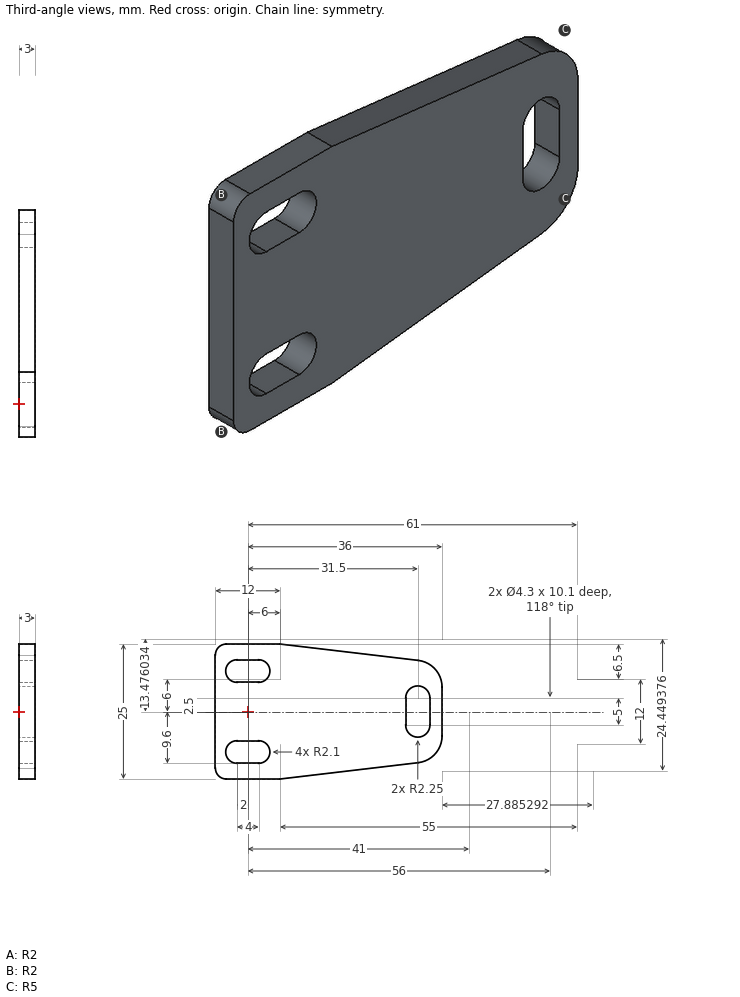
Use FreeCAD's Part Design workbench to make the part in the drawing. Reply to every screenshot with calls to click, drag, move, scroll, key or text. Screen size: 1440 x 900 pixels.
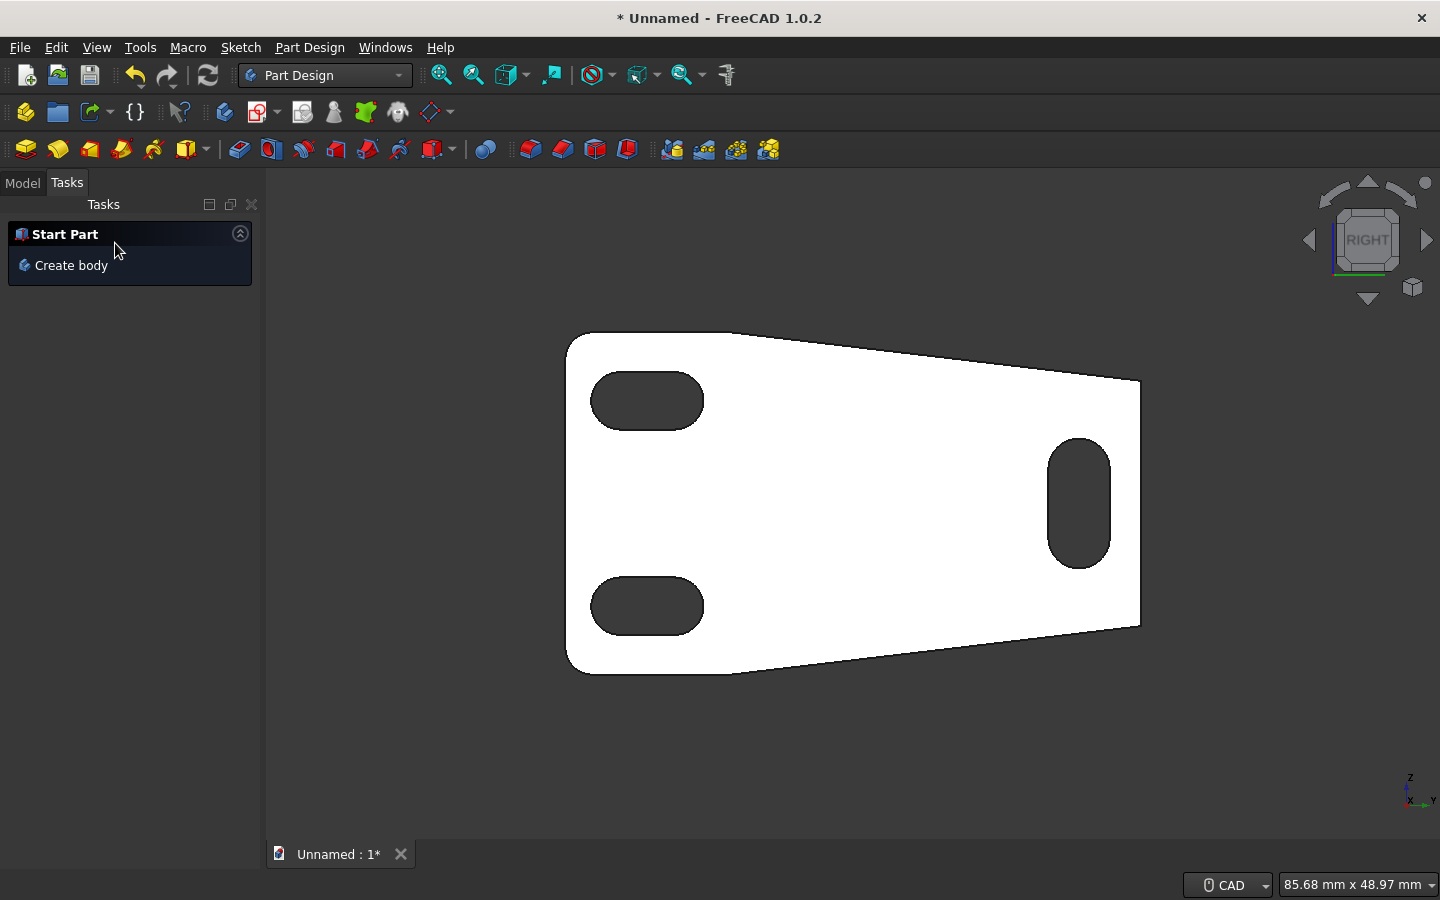
key(5)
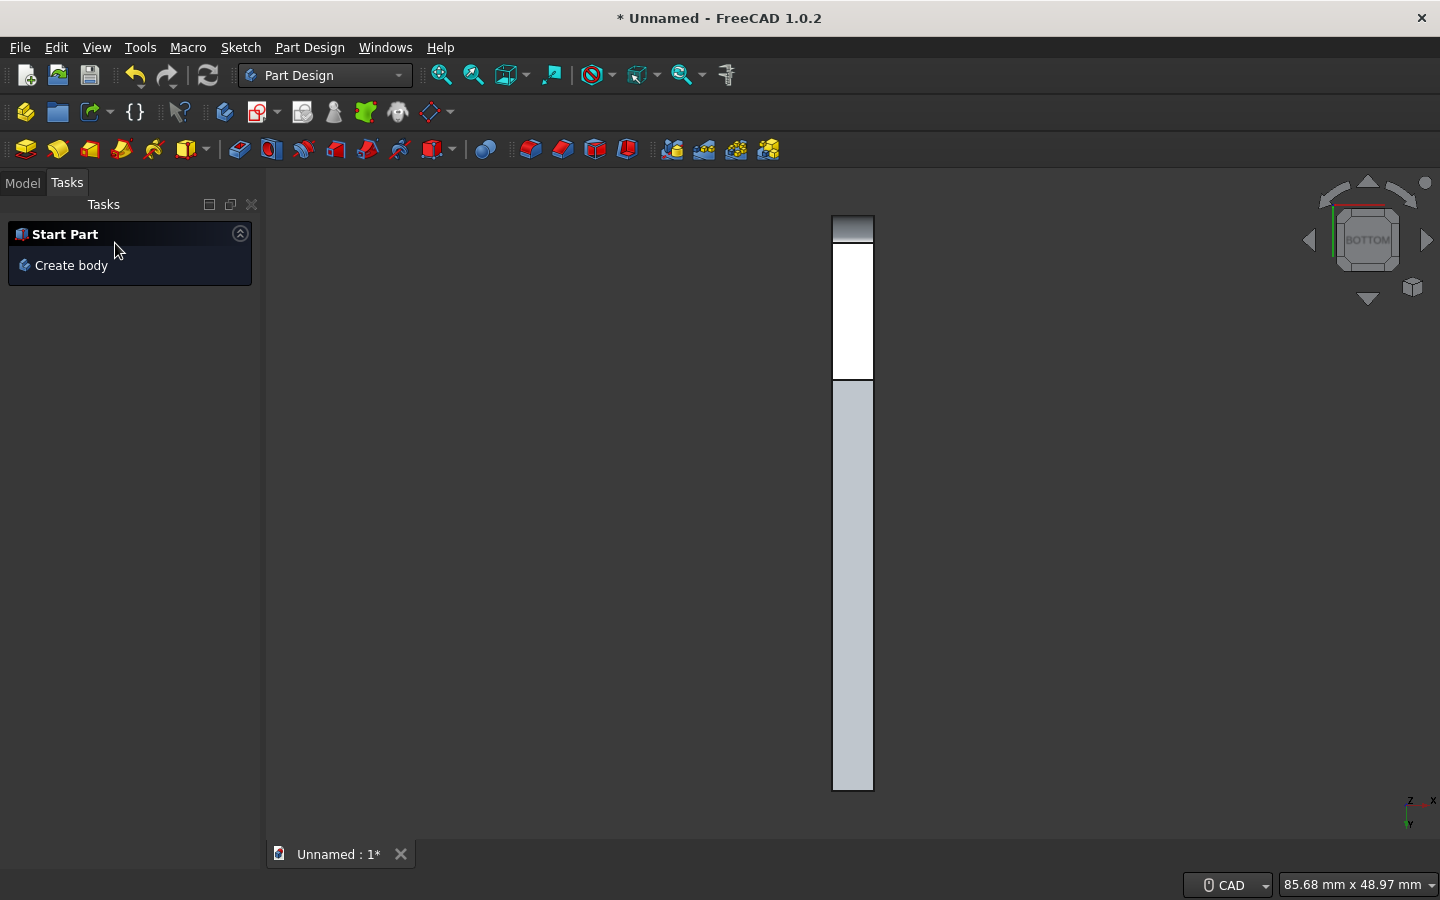
key(4)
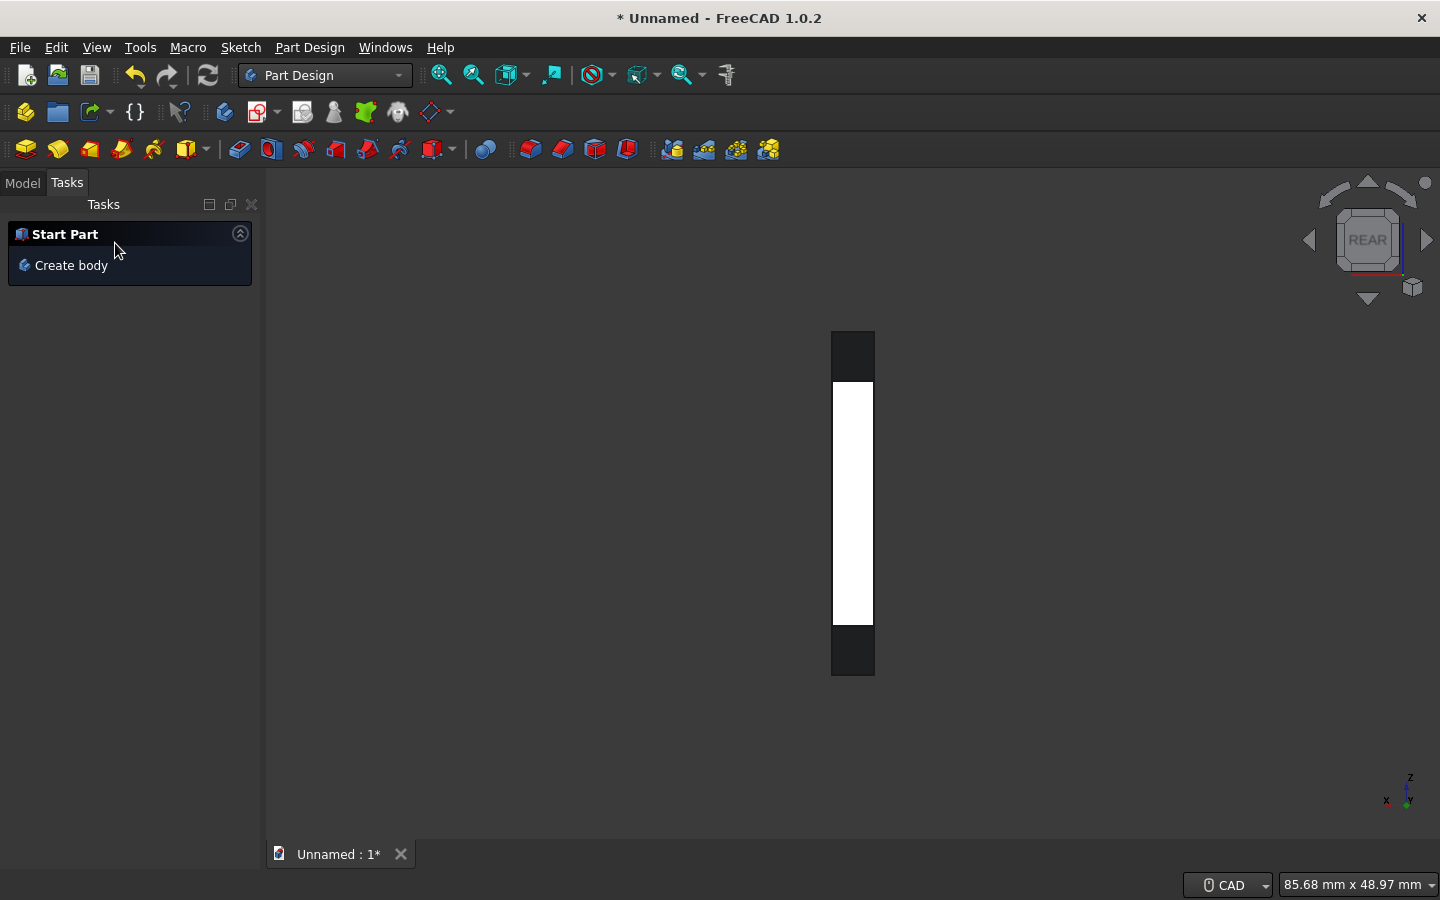
click(853, 380)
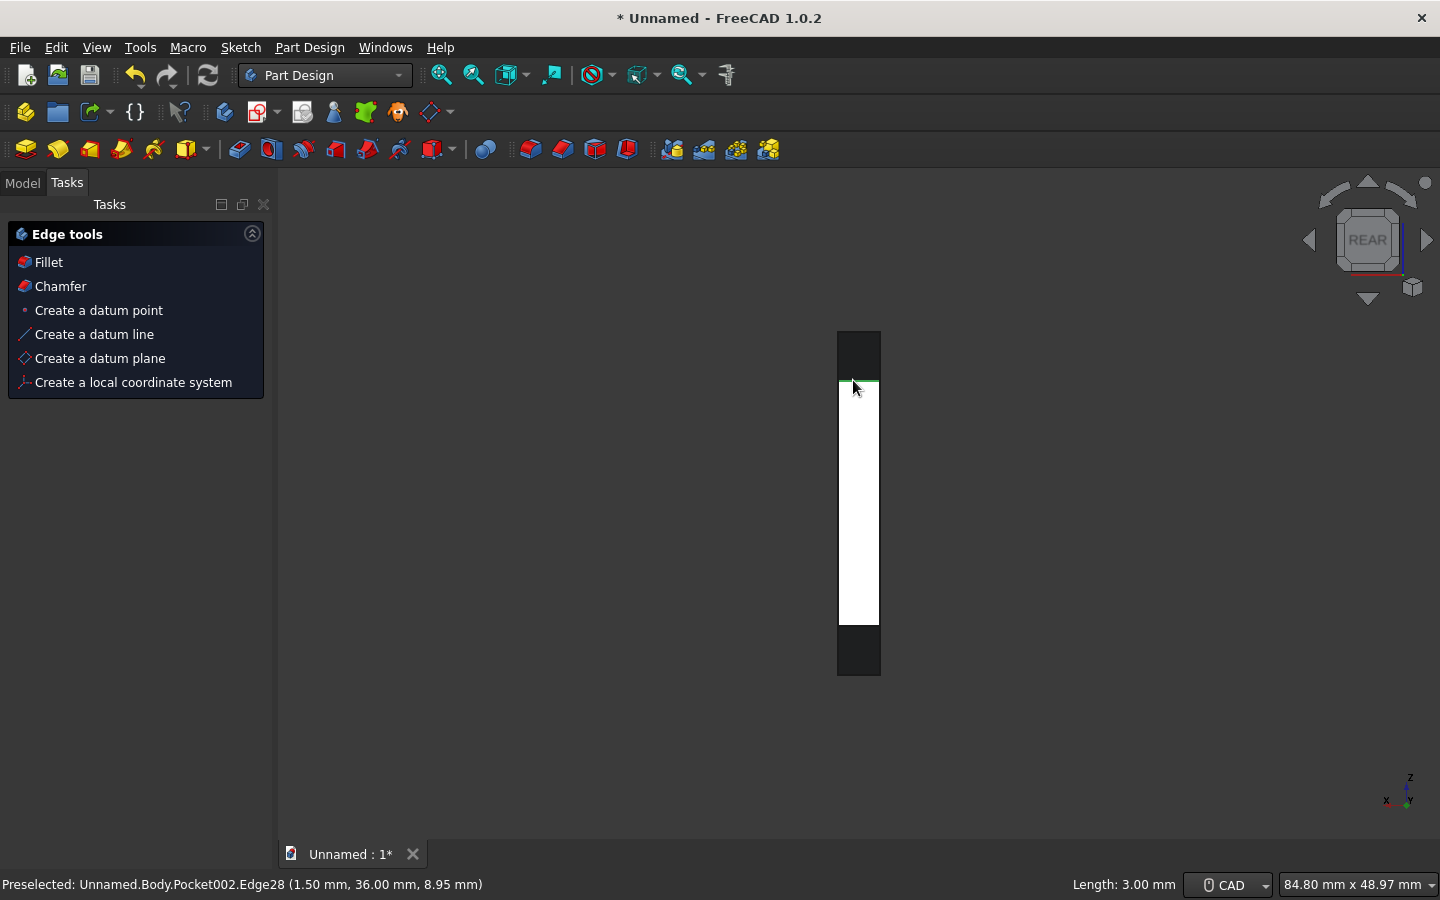
click(859, 625, ctrl)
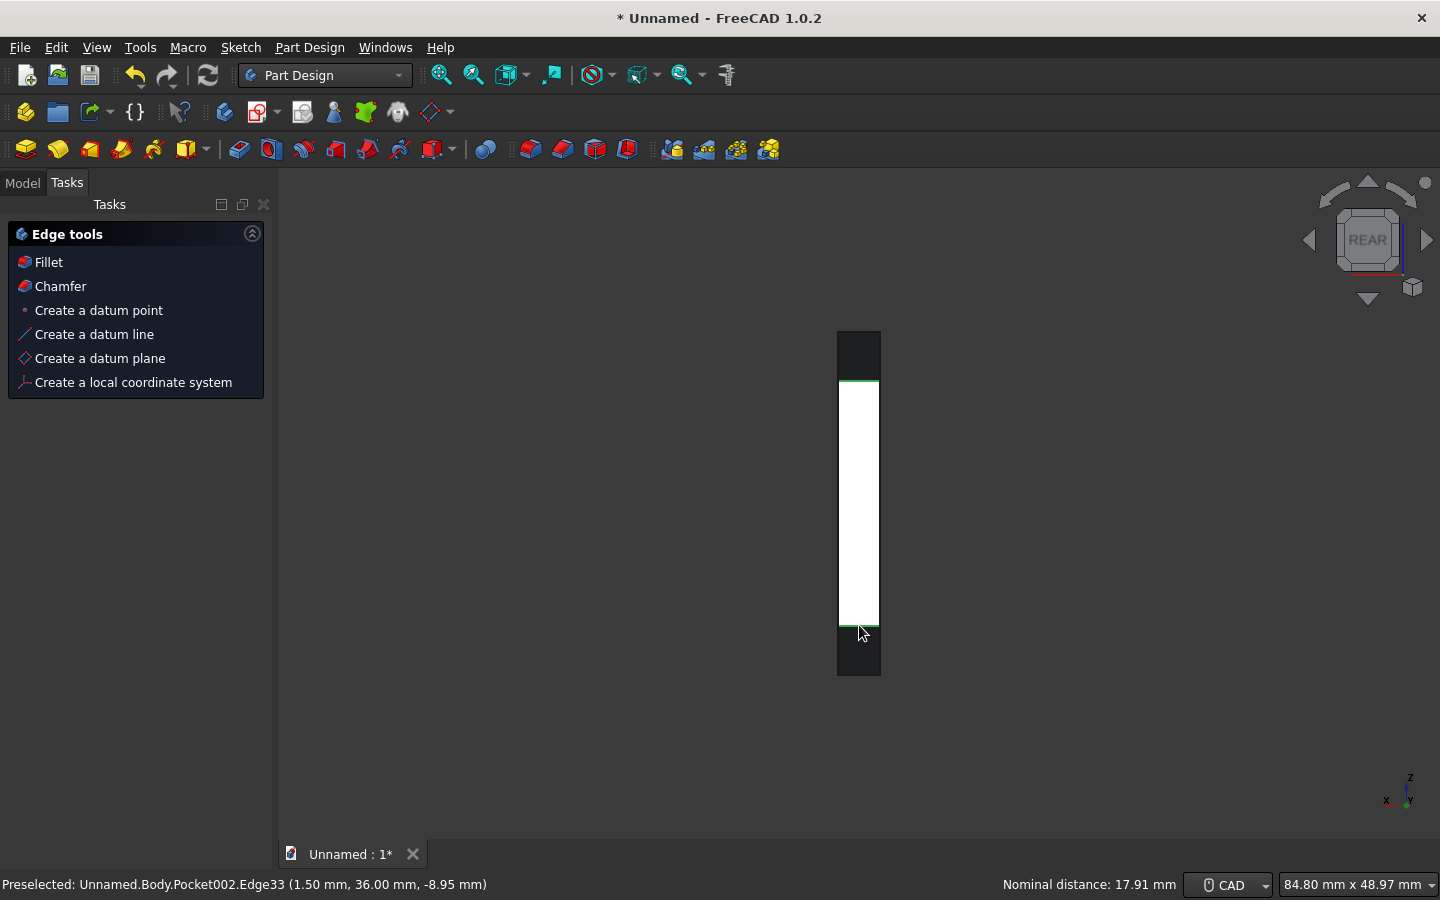
click(532, 150)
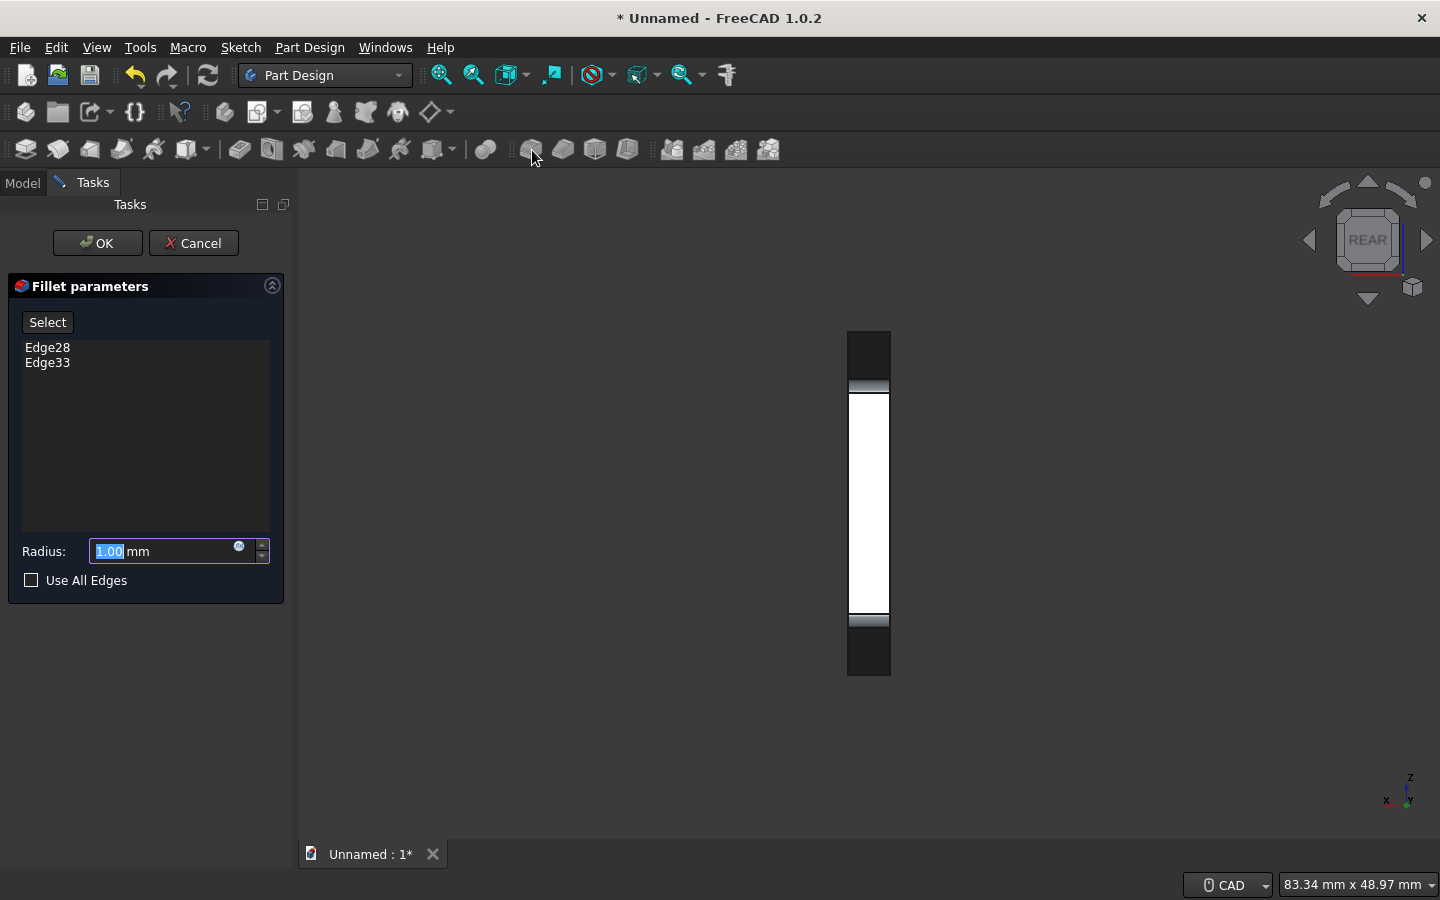
text(5)
key(Tab)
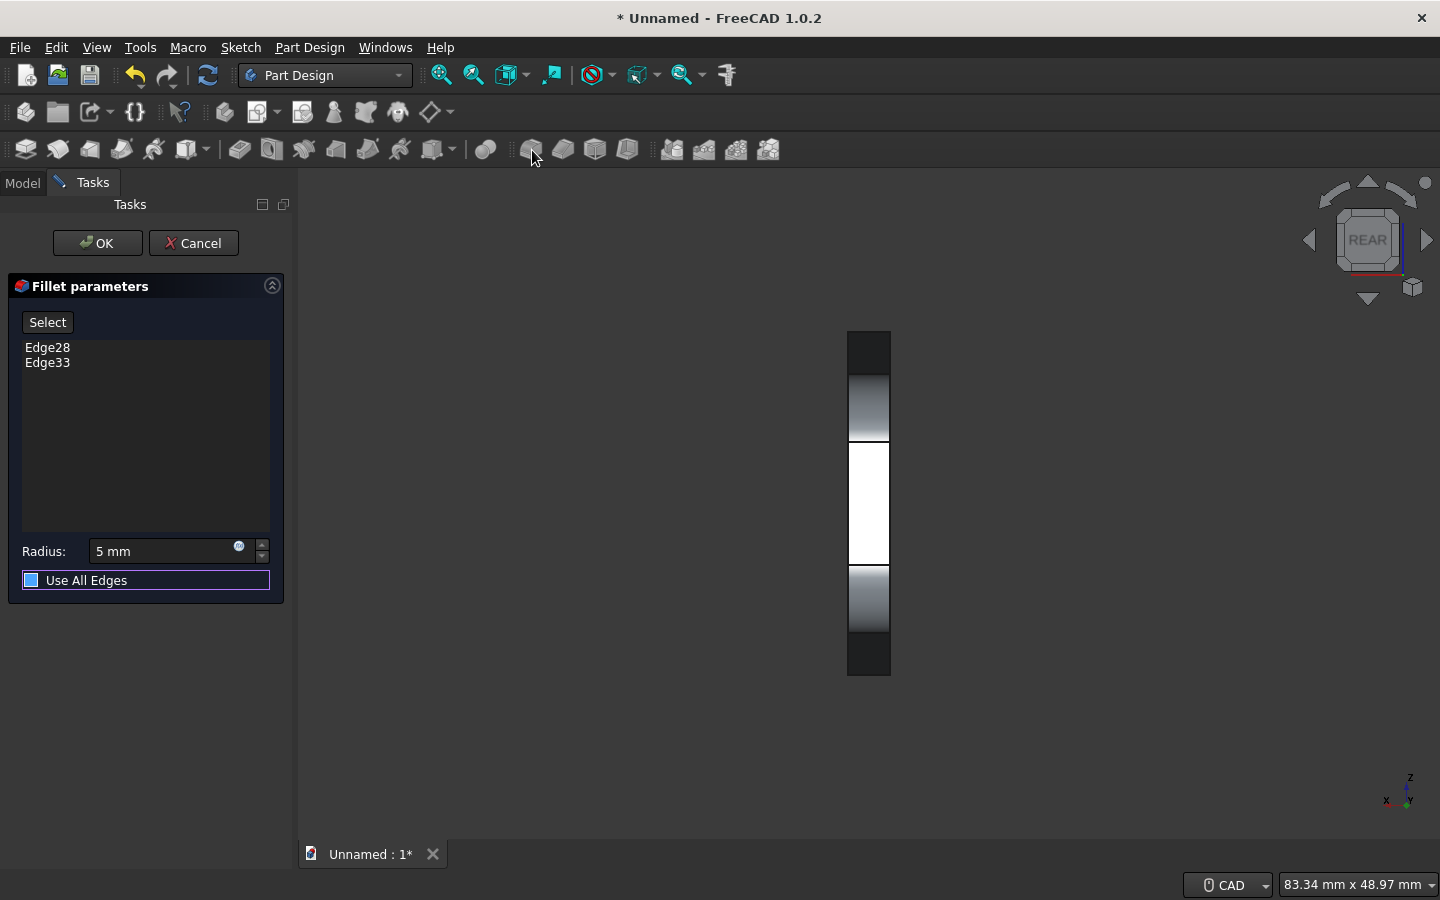
click(98, 243)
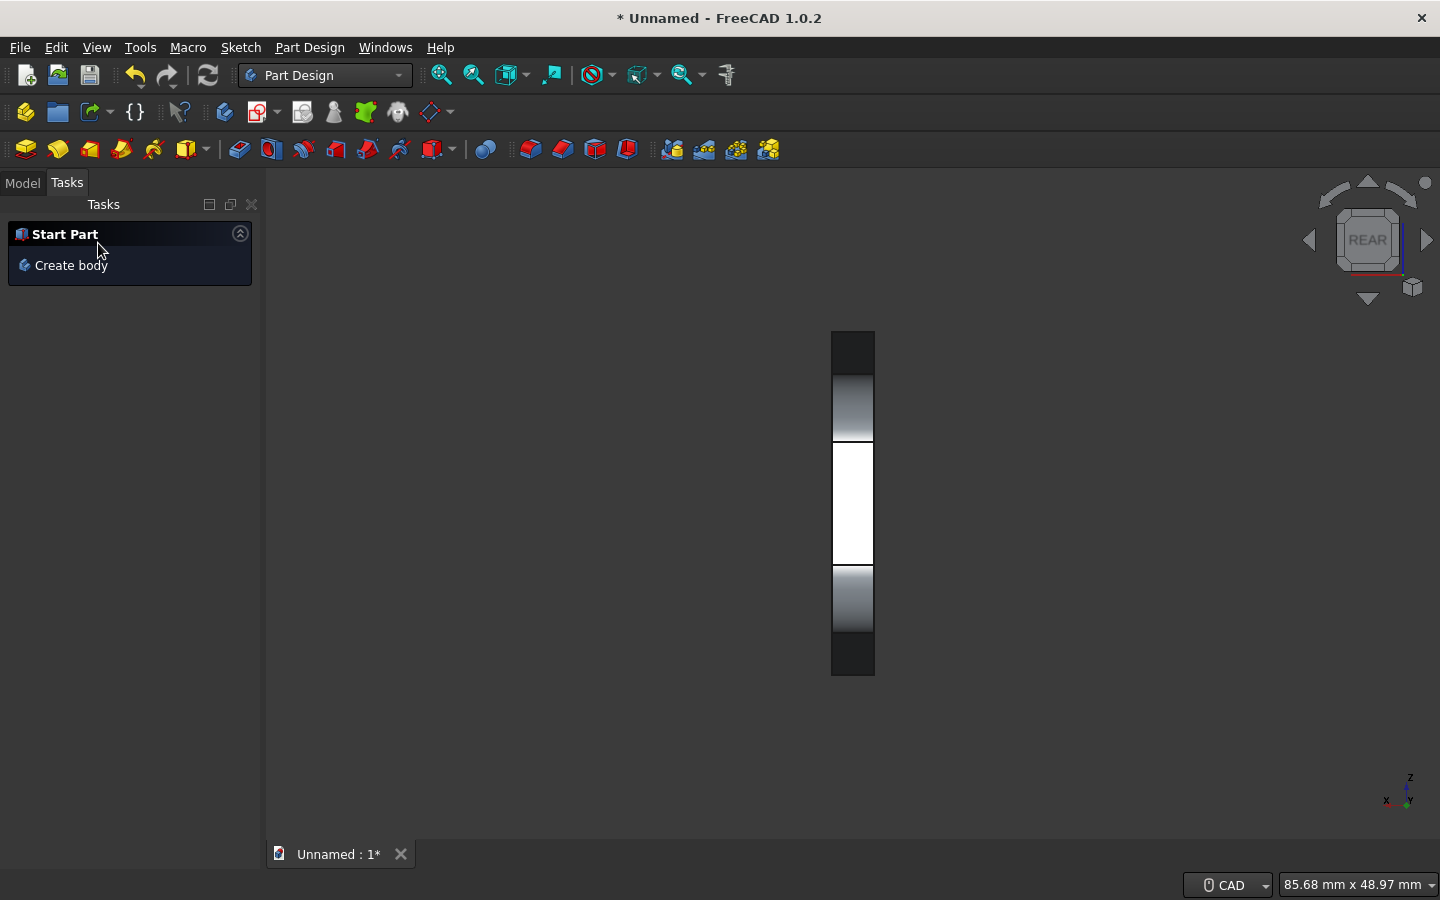
key(0)